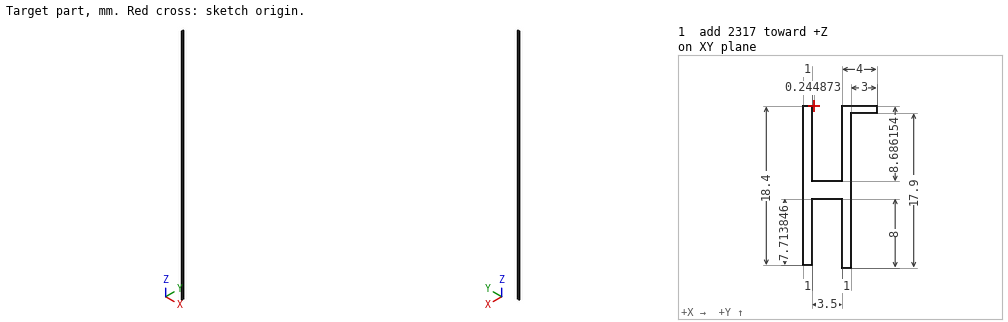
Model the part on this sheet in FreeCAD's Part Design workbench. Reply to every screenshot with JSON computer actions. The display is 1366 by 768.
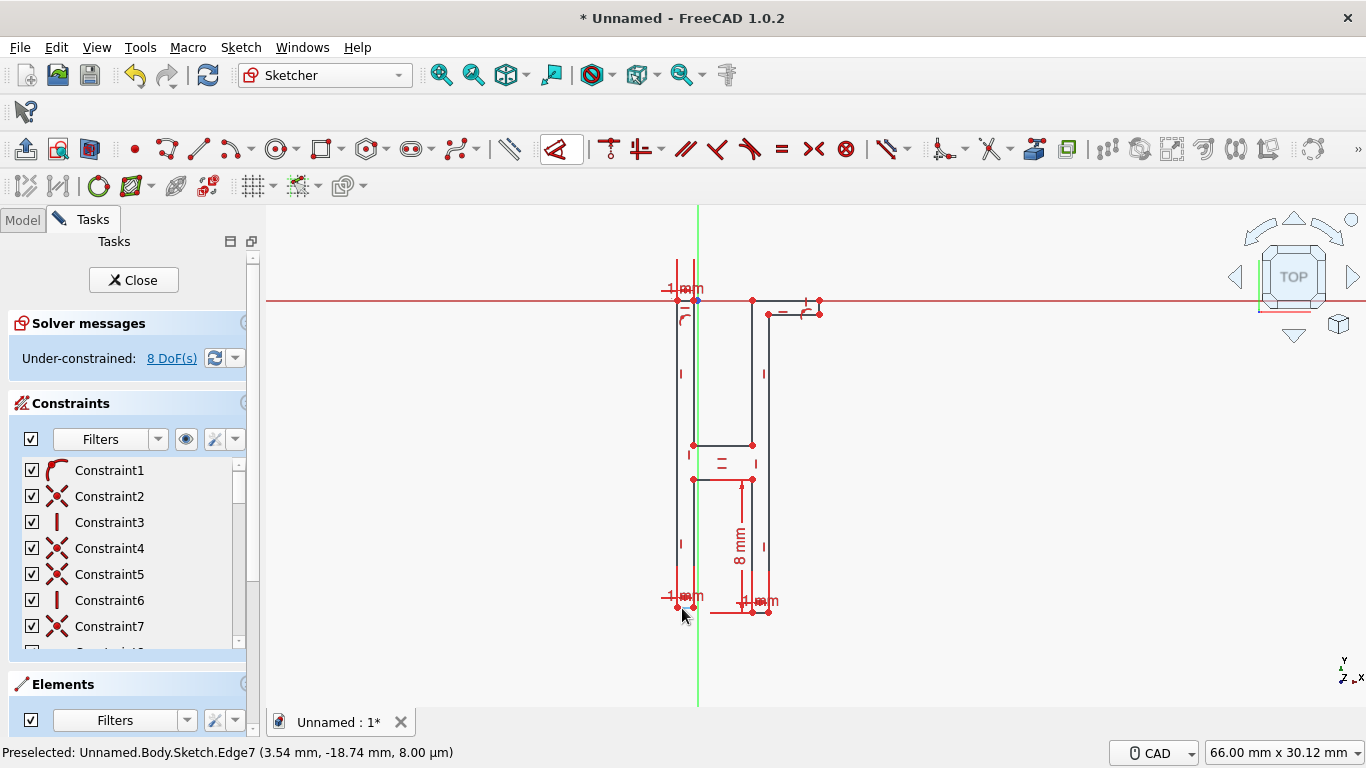
{"action": "left_click", "coordinate": [799, 315]}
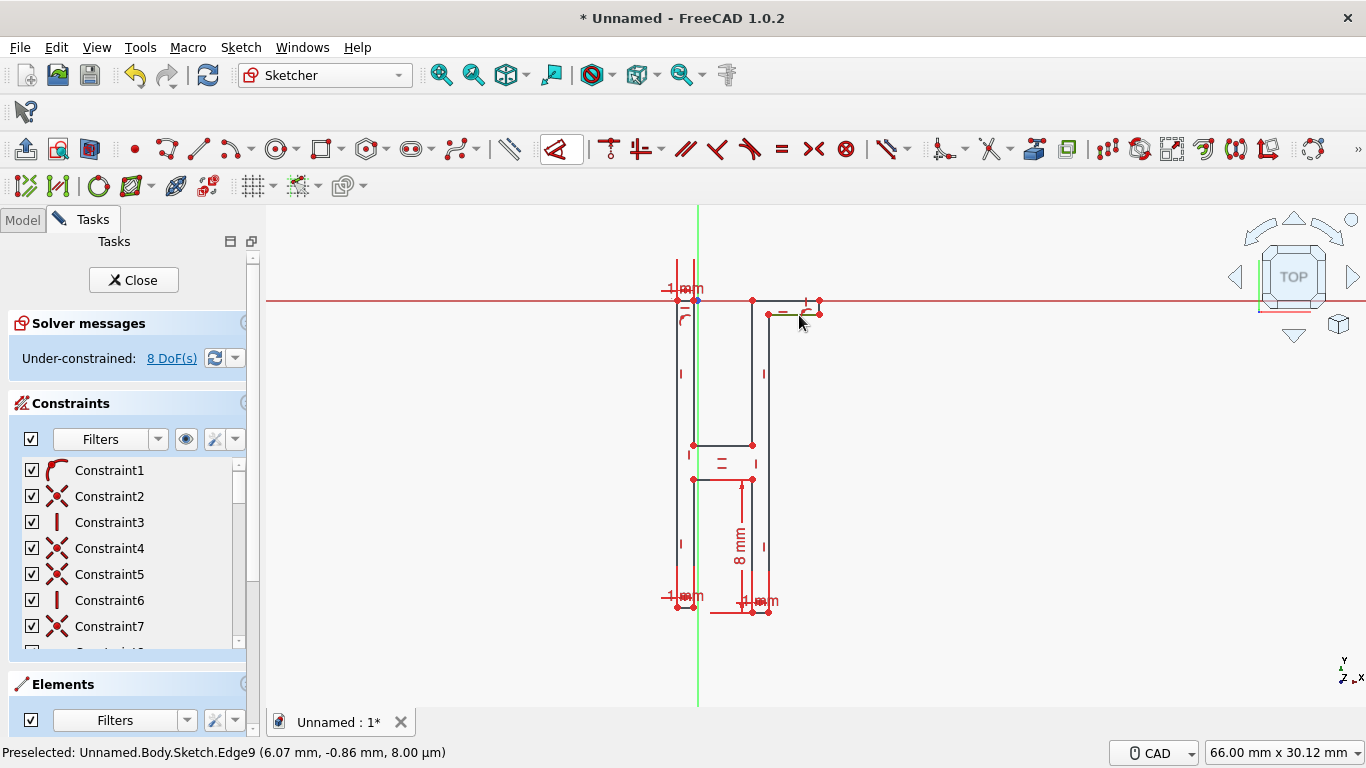
{"action": "left_click", "coordinate": [578, 150]}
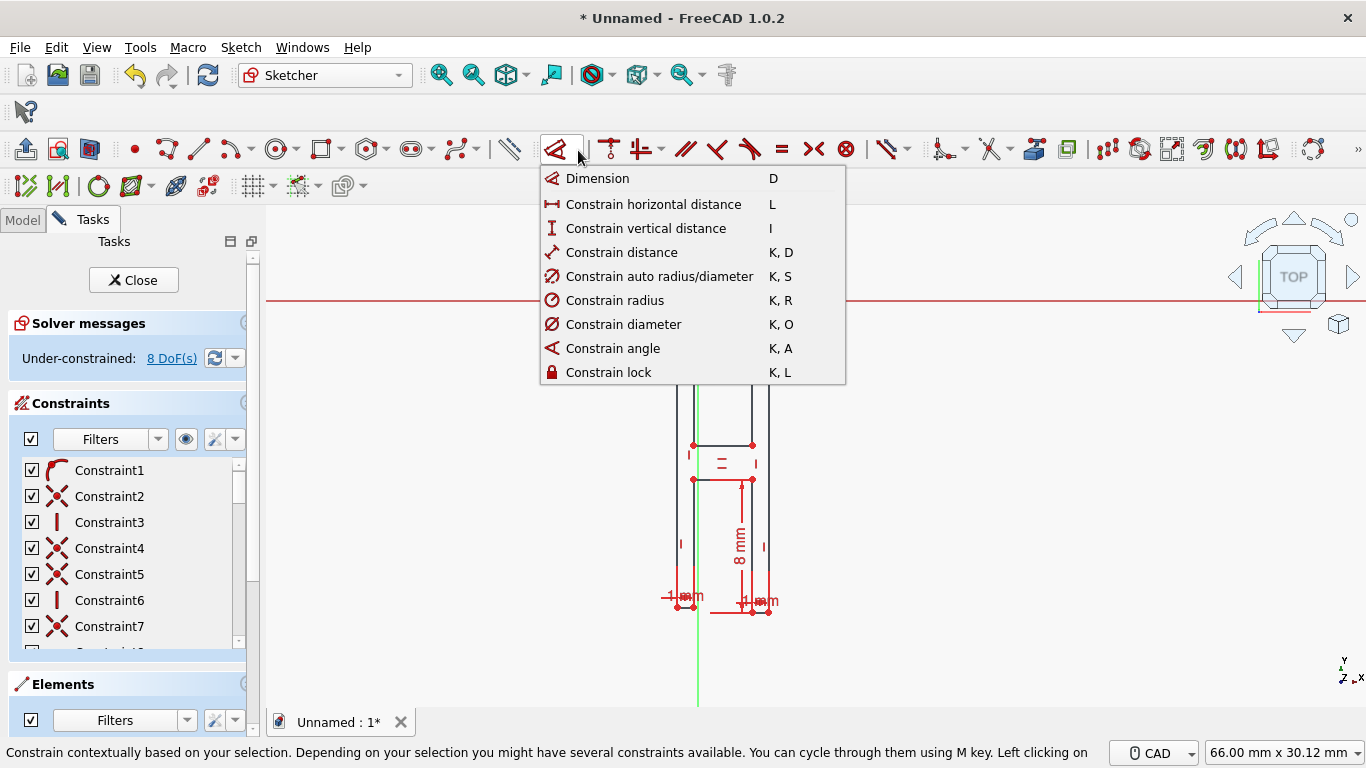
{"action": "left_click", "coordinate": [693, 204]}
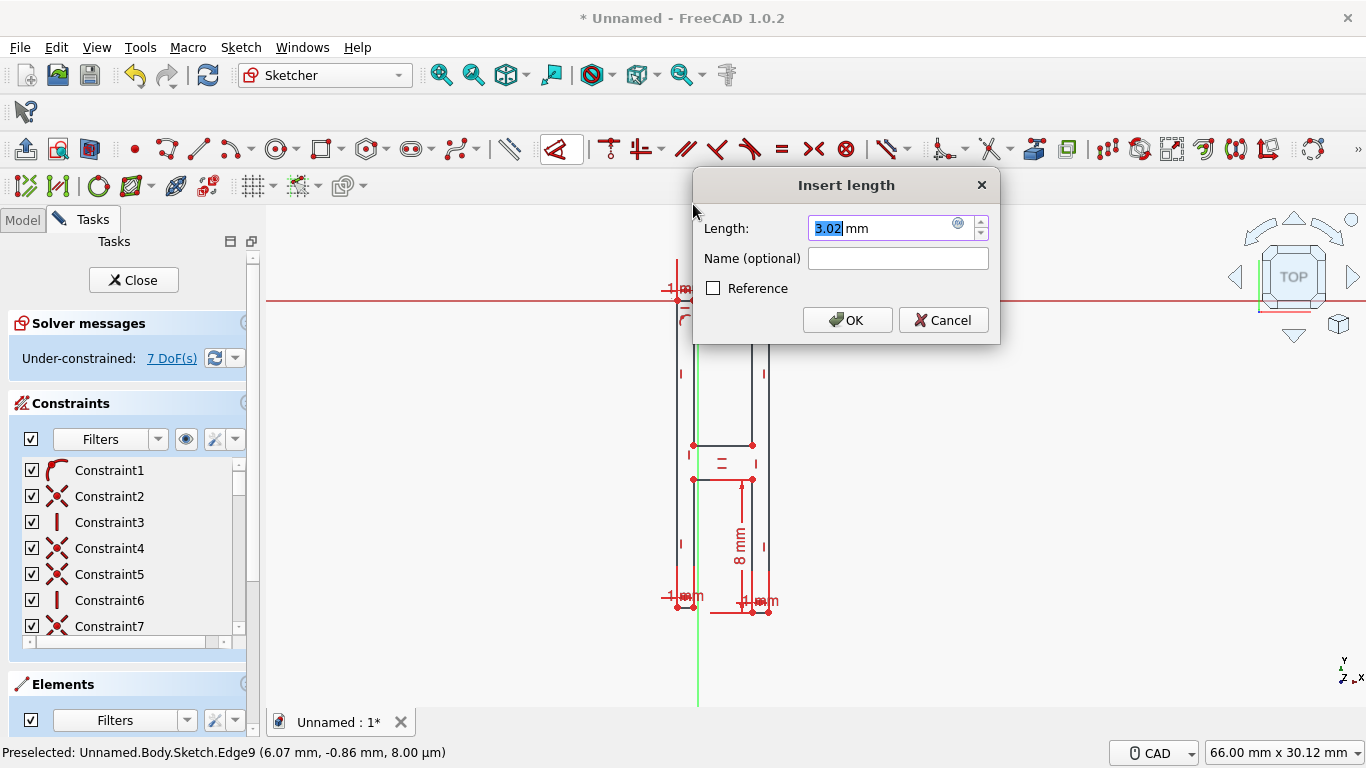
{"action": "type", "text": "3"}
{"action": "key", "text": "Return"}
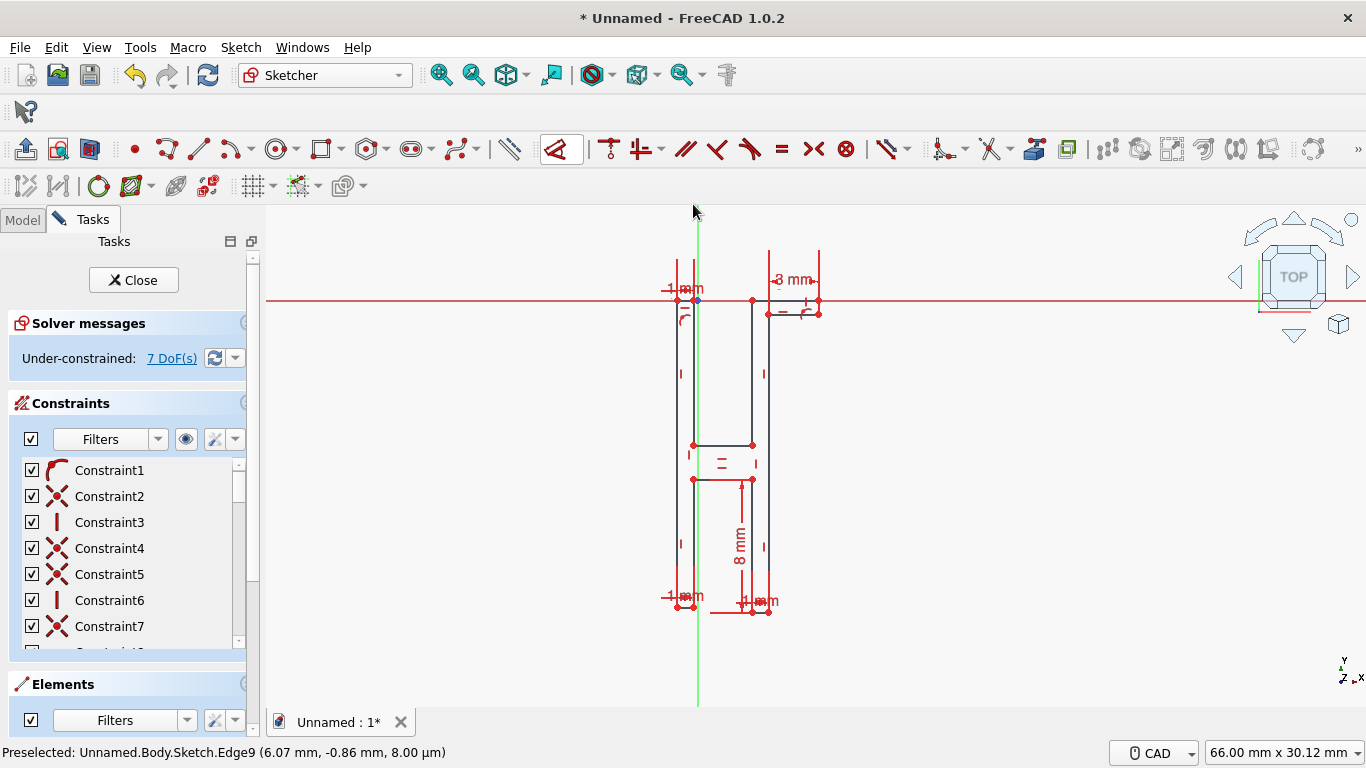
{"action": "left_click", "coordinate": [799, 301]}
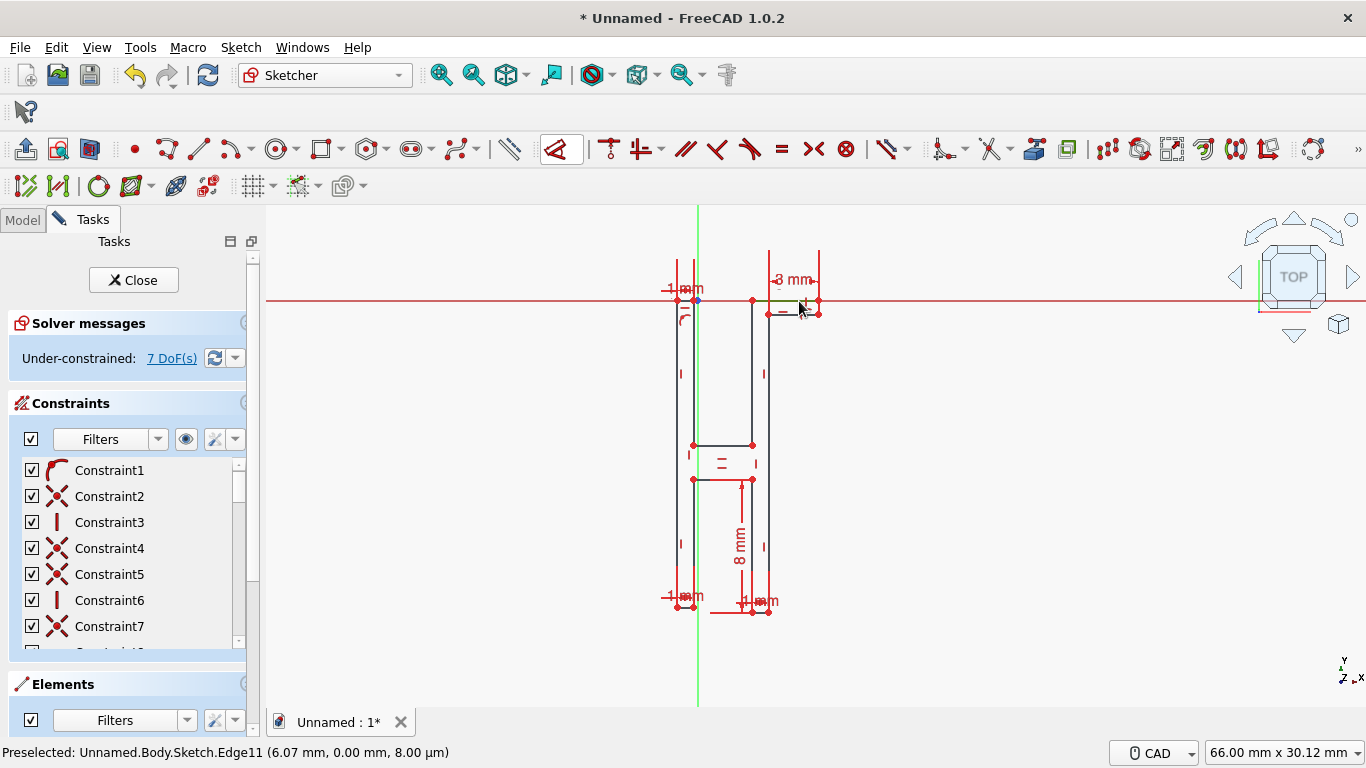
{"action": "left_click", "coordinate": [578, 150]}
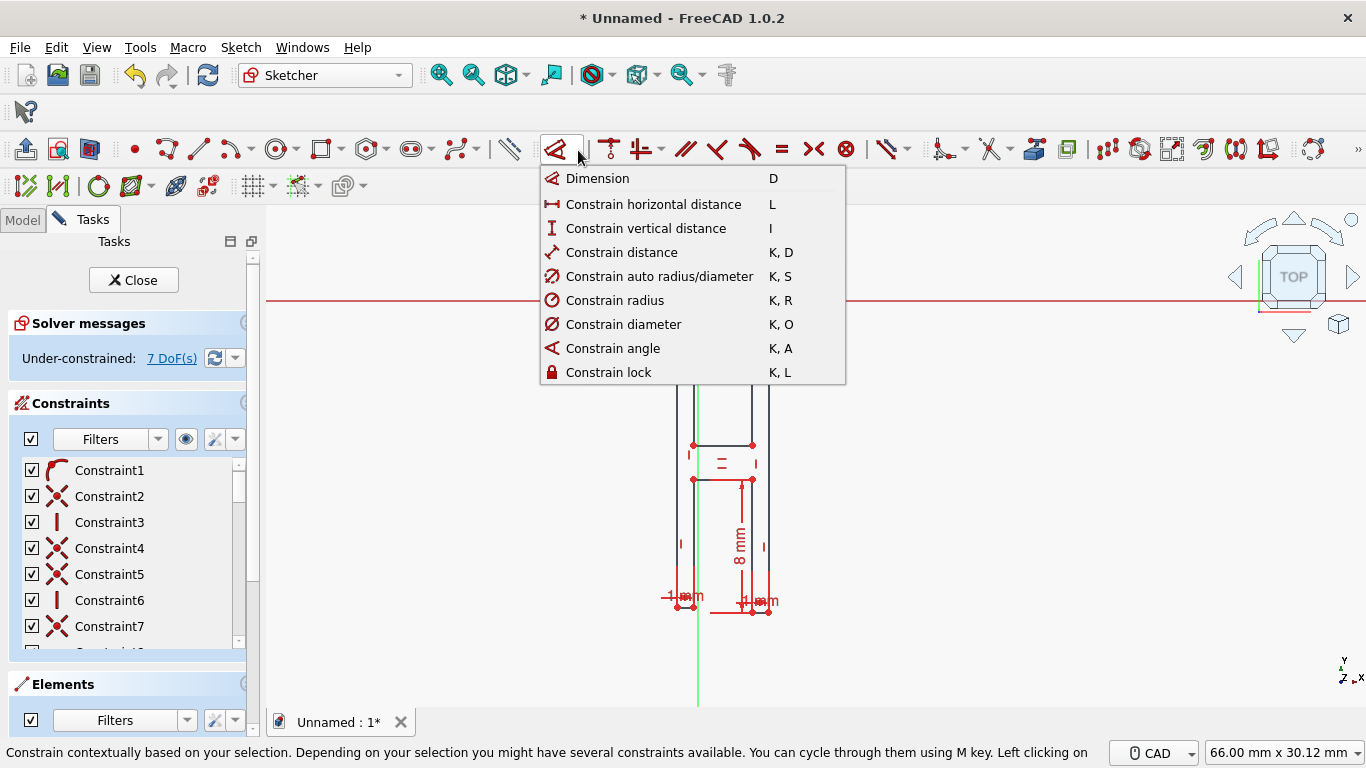
{"action": "left_click", "coordinate": [693, 204]}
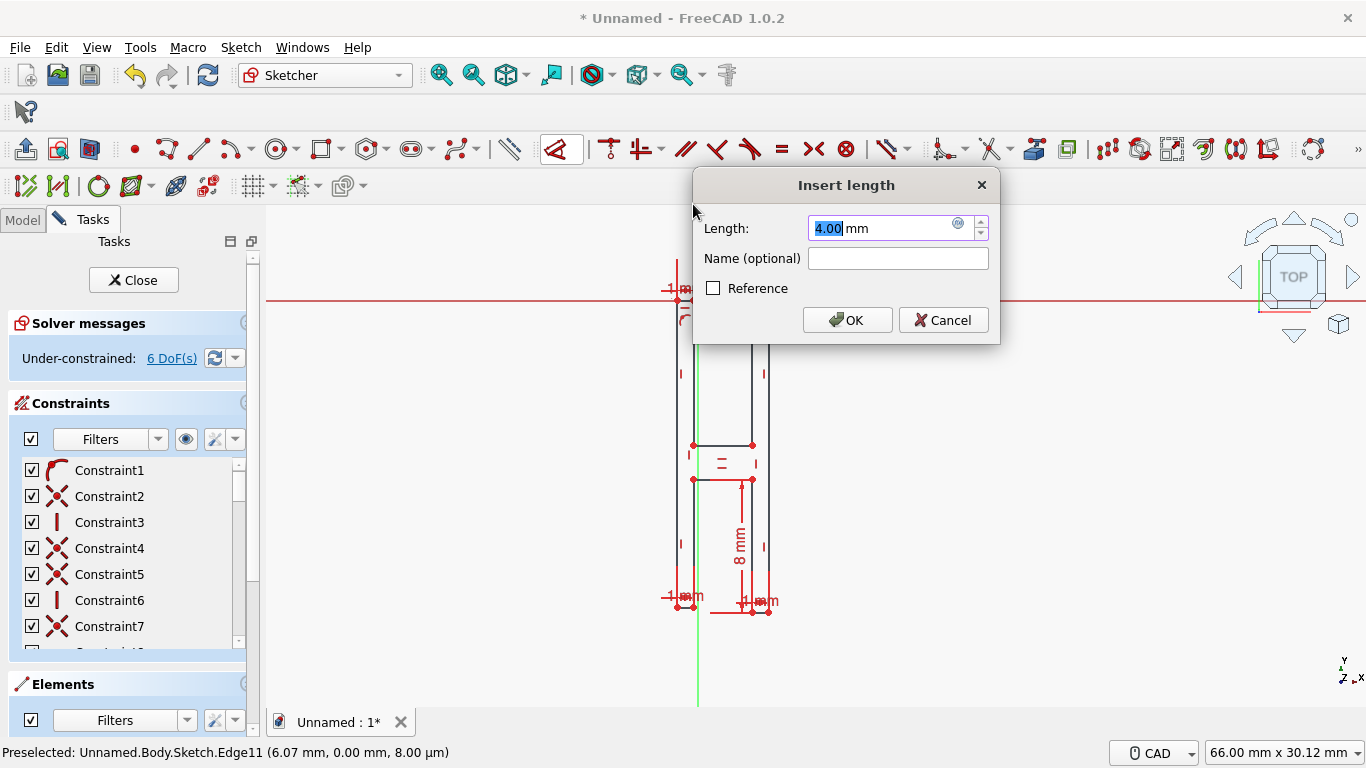
{"action": "type", "text": "4"}
{"action": "key", "text": "Return"}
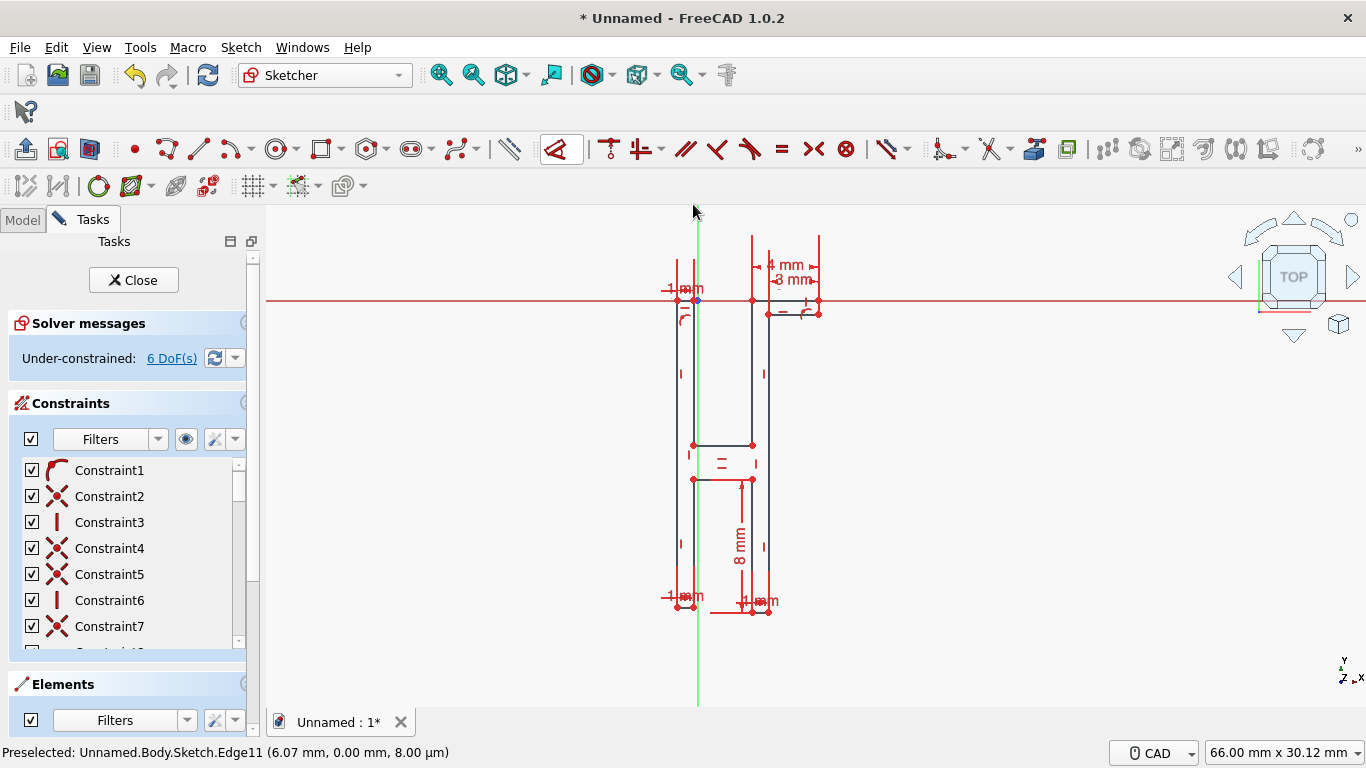
{"action": "left_click", "coordinate": [711, 480]}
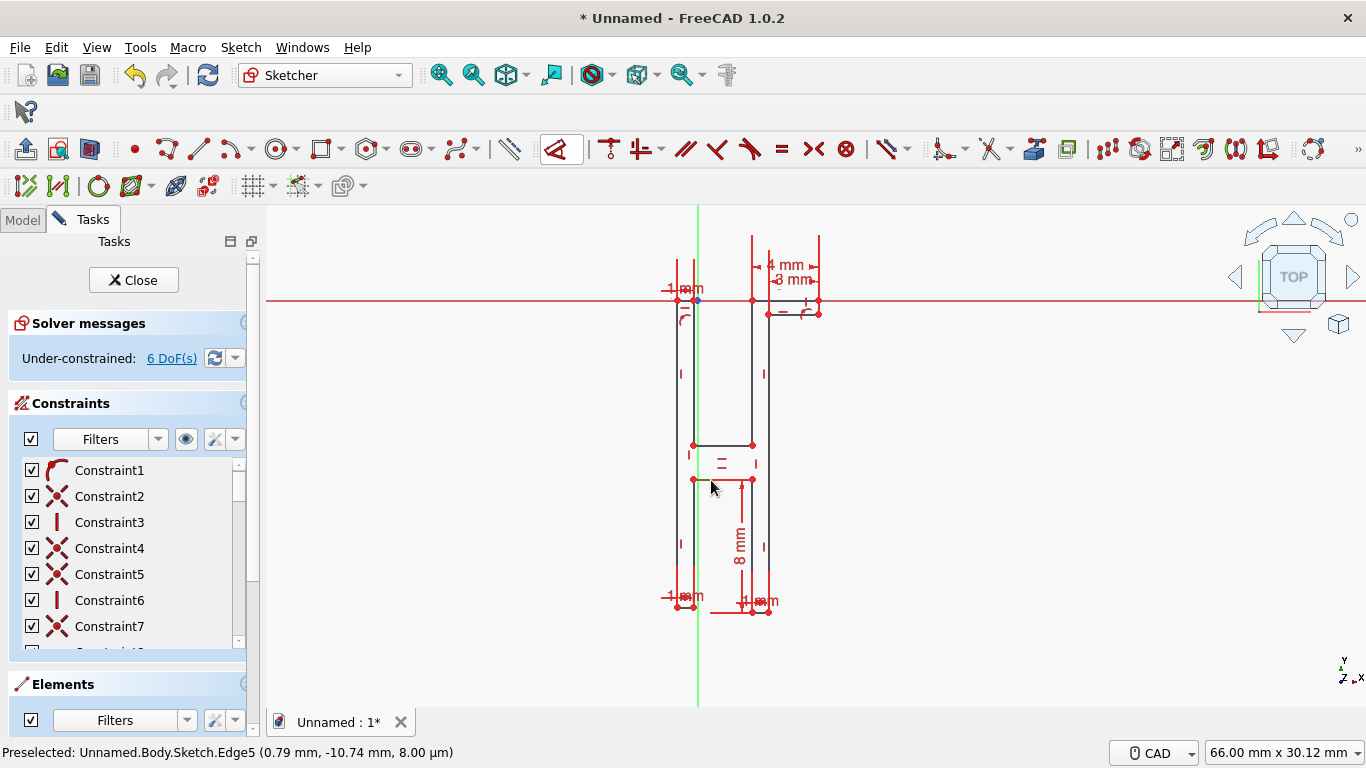
{"action": "key", "text": "l"}